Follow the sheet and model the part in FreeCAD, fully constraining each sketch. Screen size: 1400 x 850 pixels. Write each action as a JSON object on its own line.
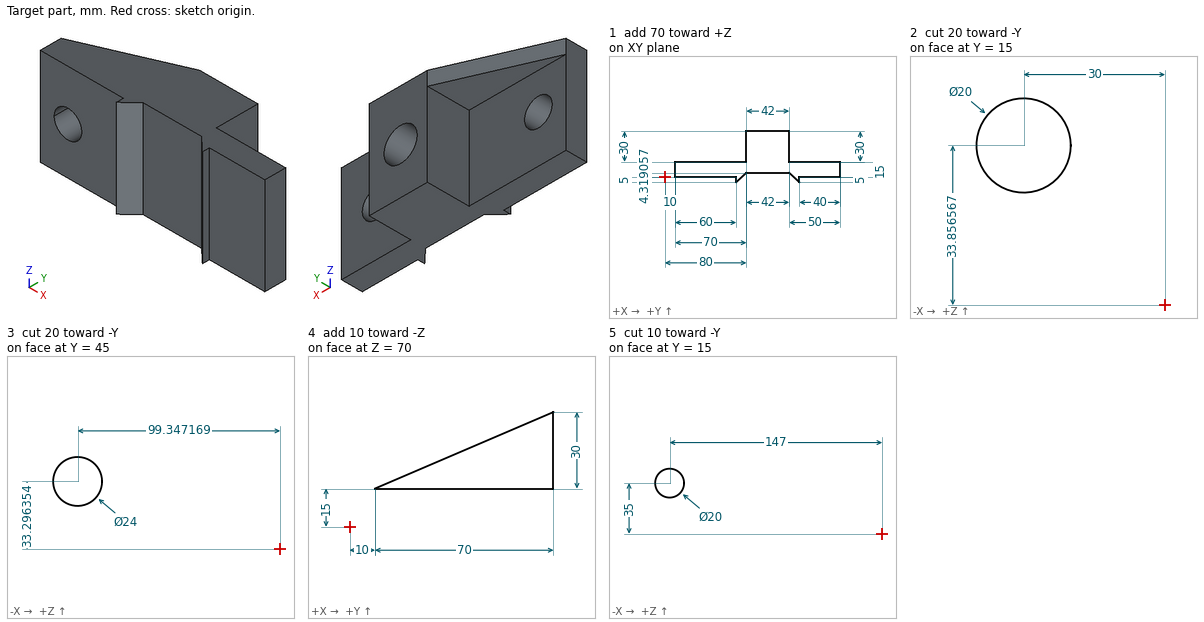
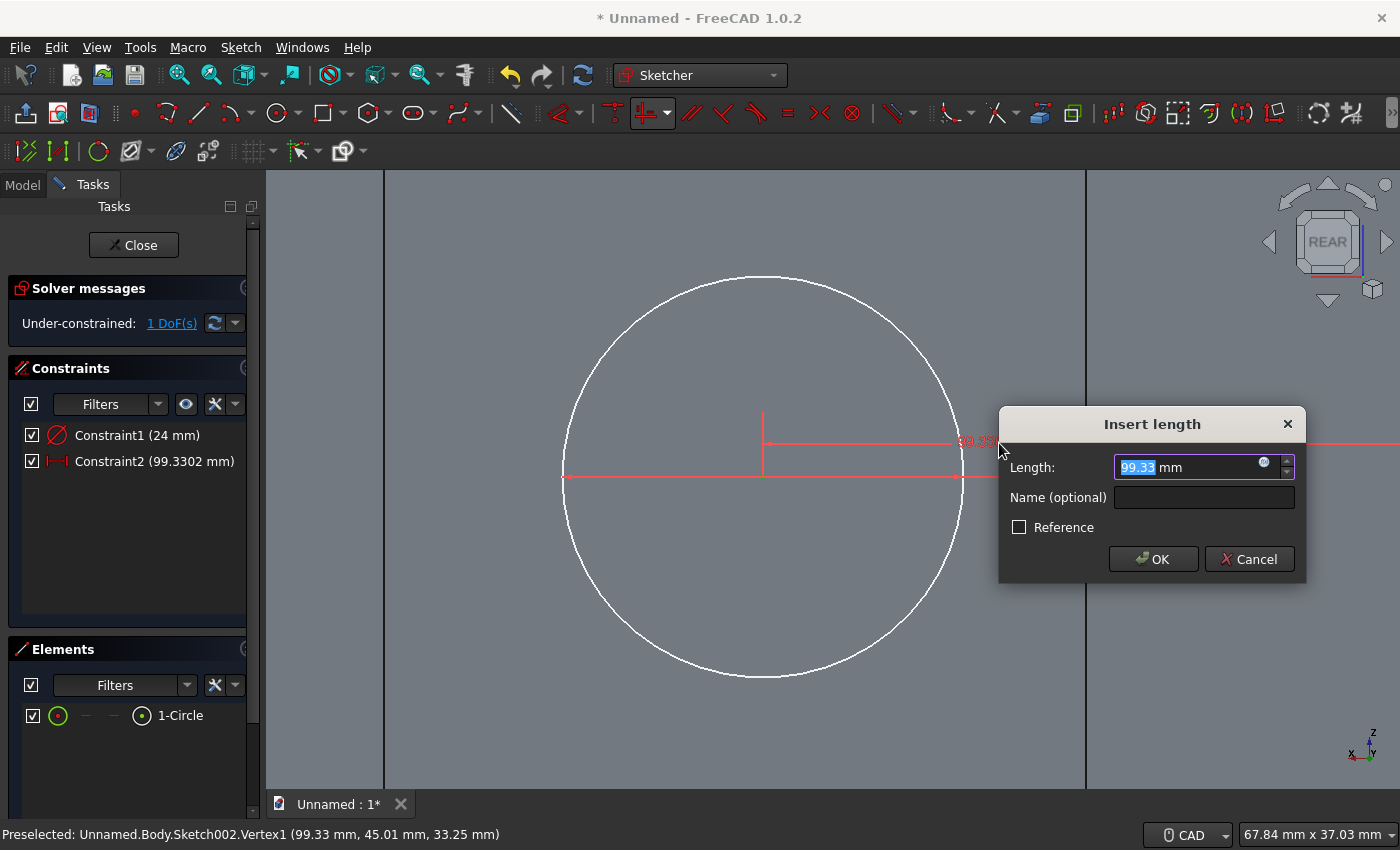
{"action": "type", "text": "99.347169"}
{"action": "key", "text": "Return"}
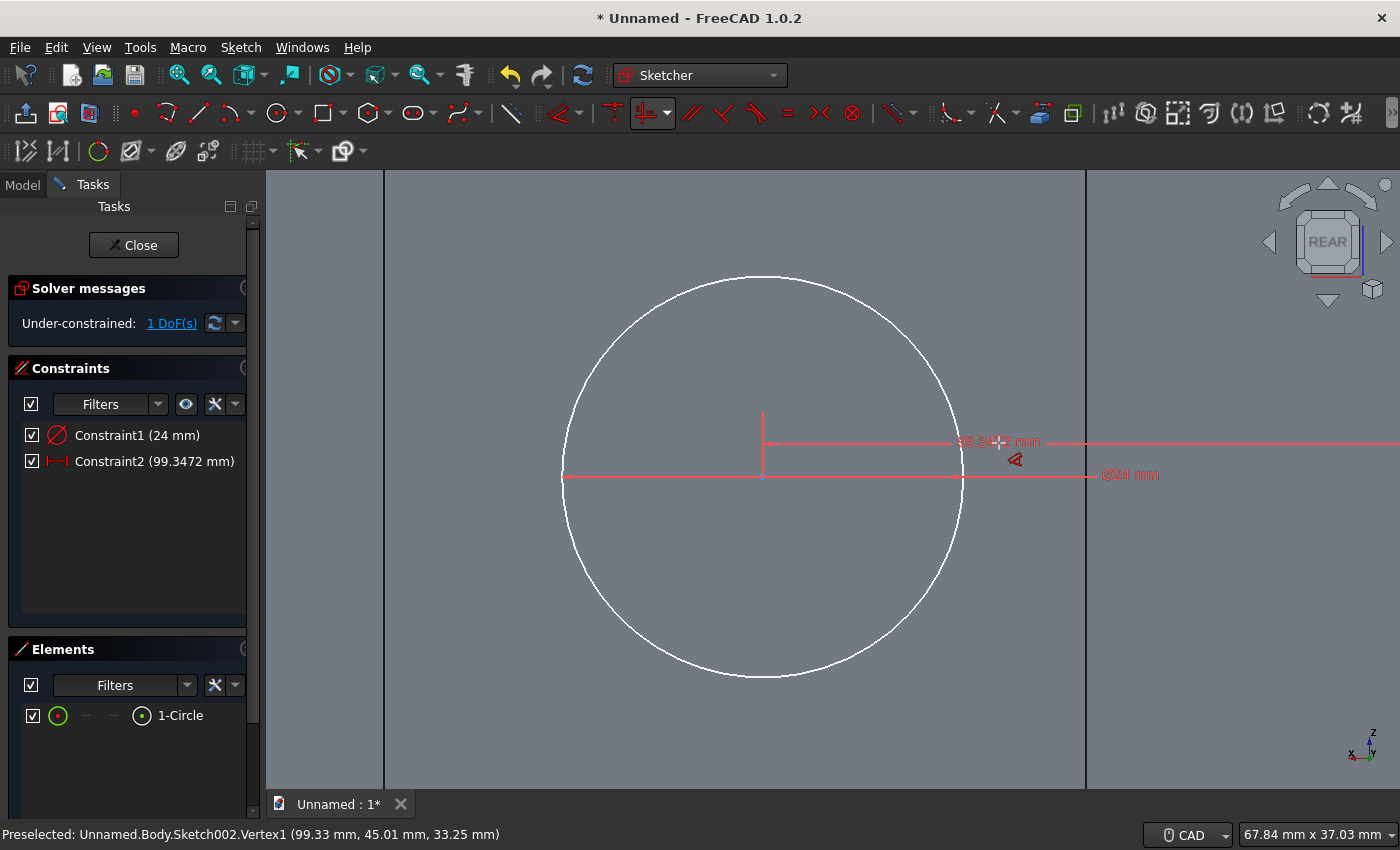
{"action": "left_click", "coordinate": [763, 477]}
{"action": "left_click", "coordinate": [729, 619]}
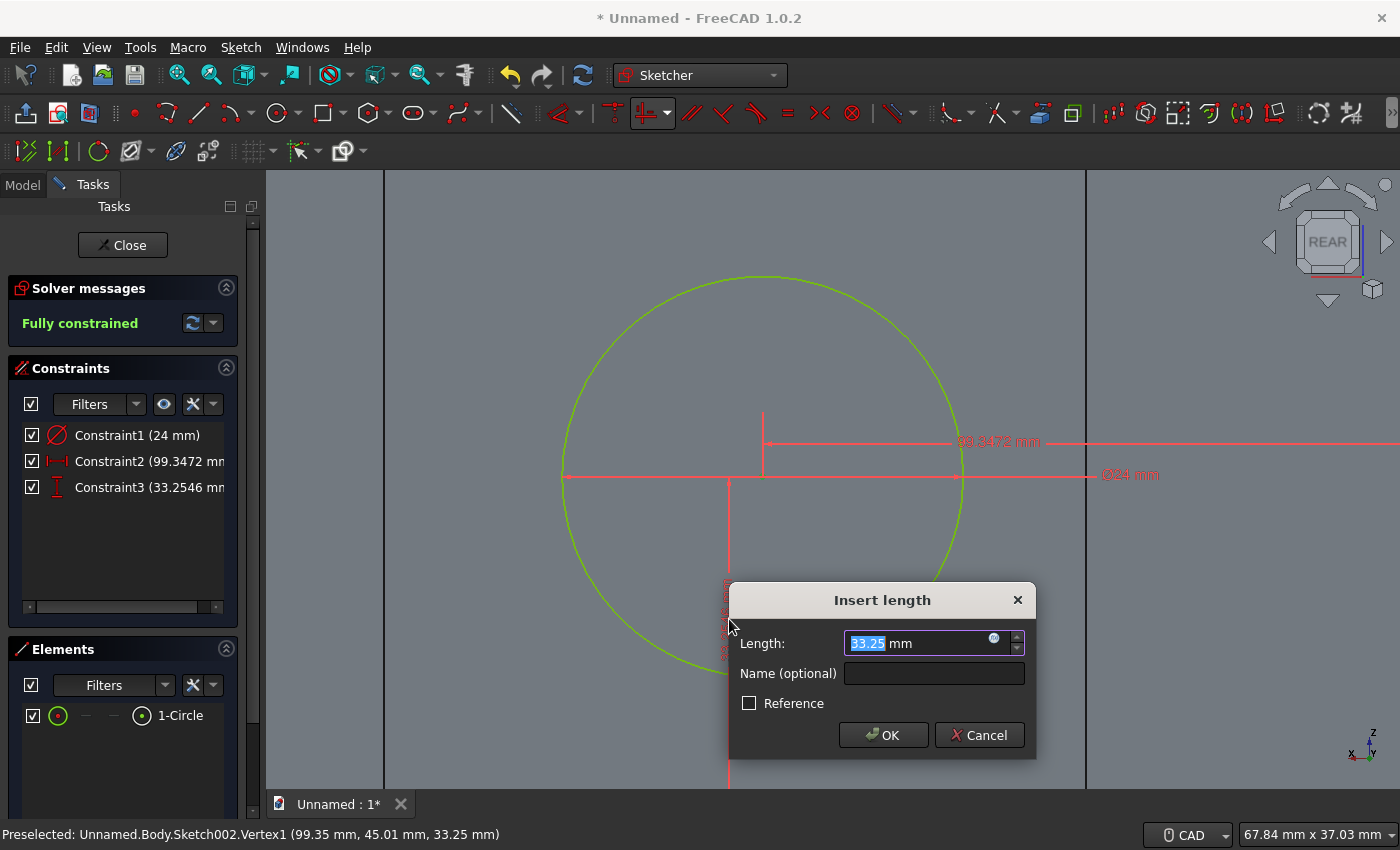
{"action": "type", "text": "33.296354"}
{"action": "key", "text": "Return"}
{"action": "key", "text": "Escape"}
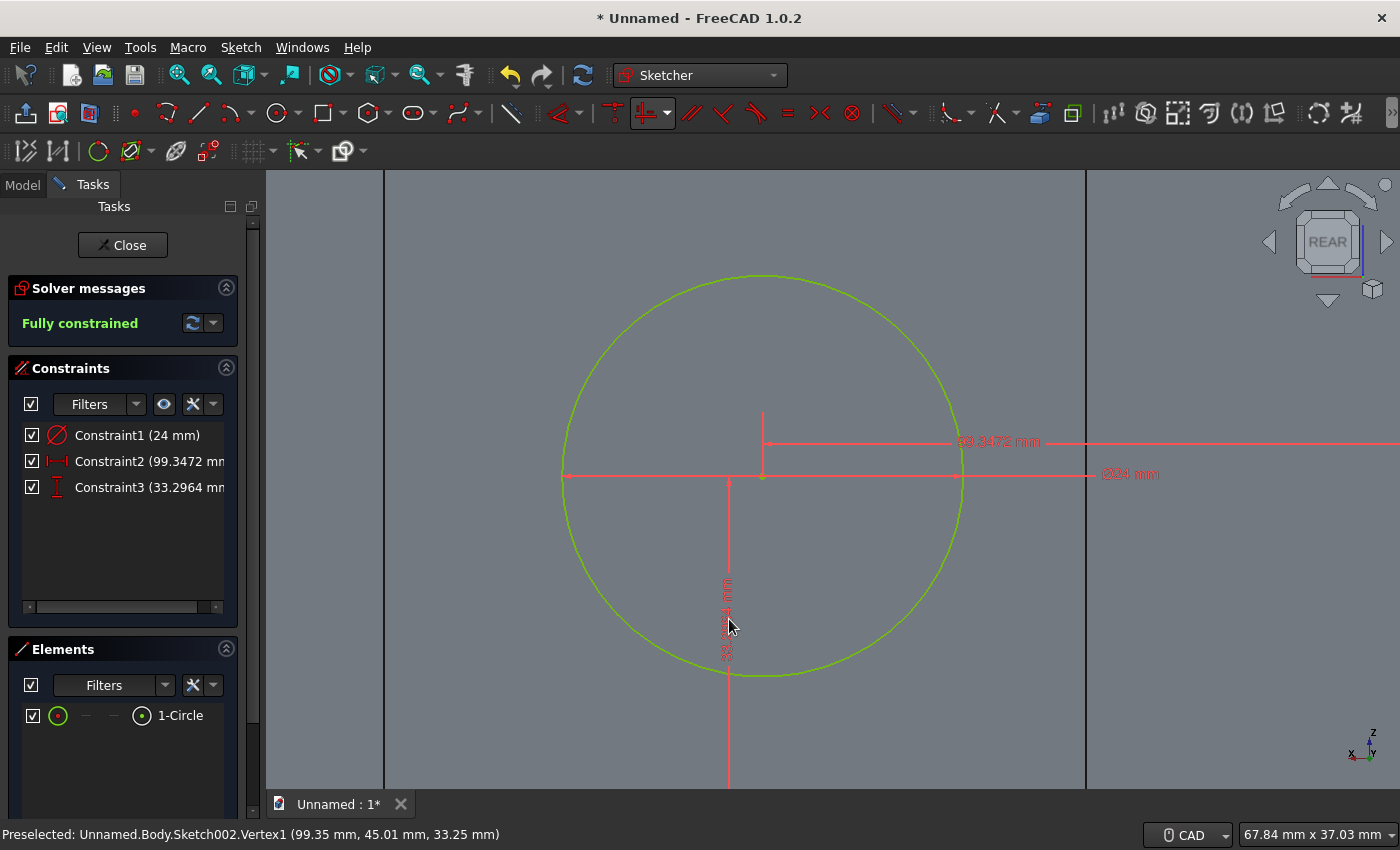
{"action": "left_click", "coordinate": [123, 245]}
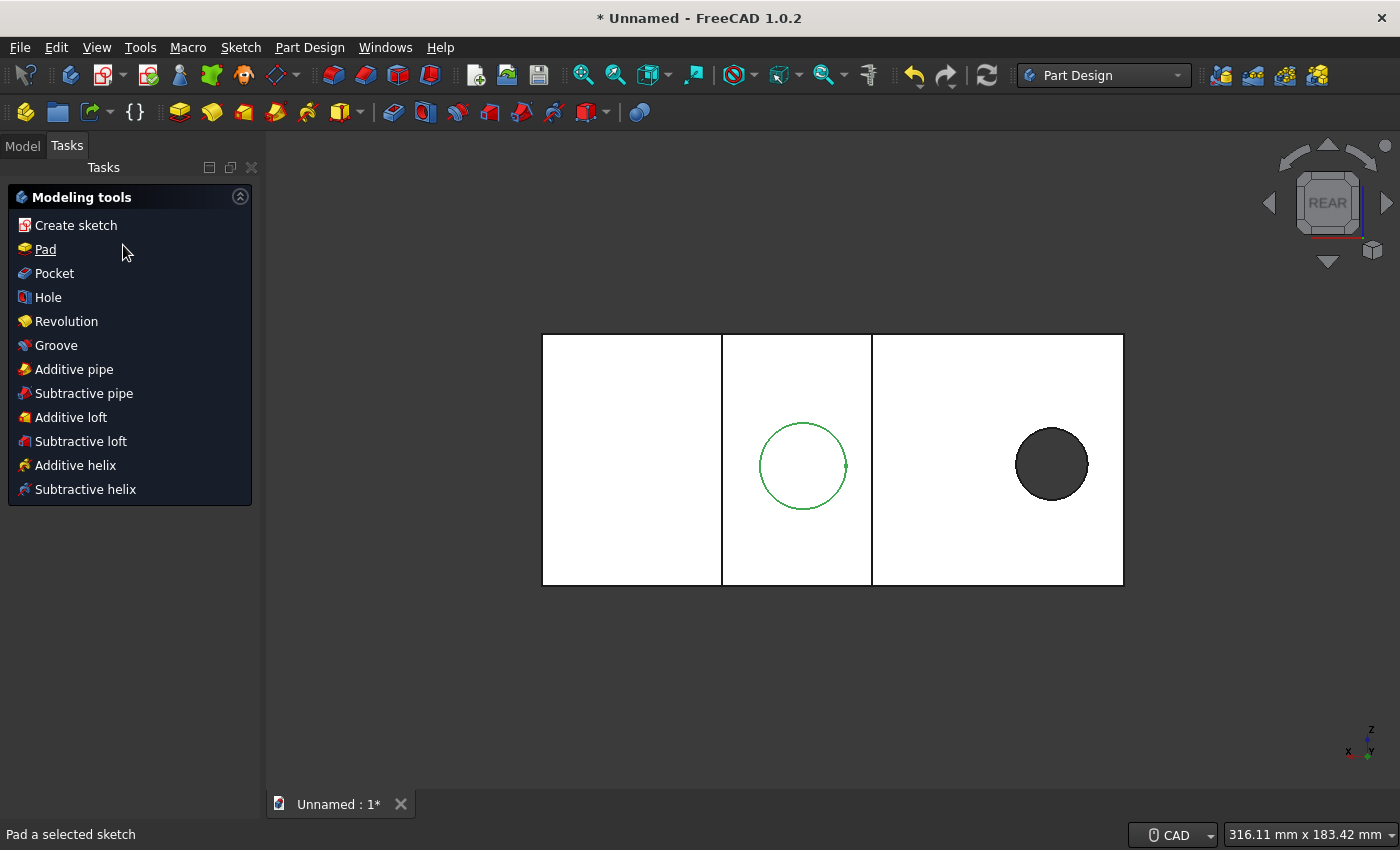
{"action": "left_click", "coordinate": [394, 112]}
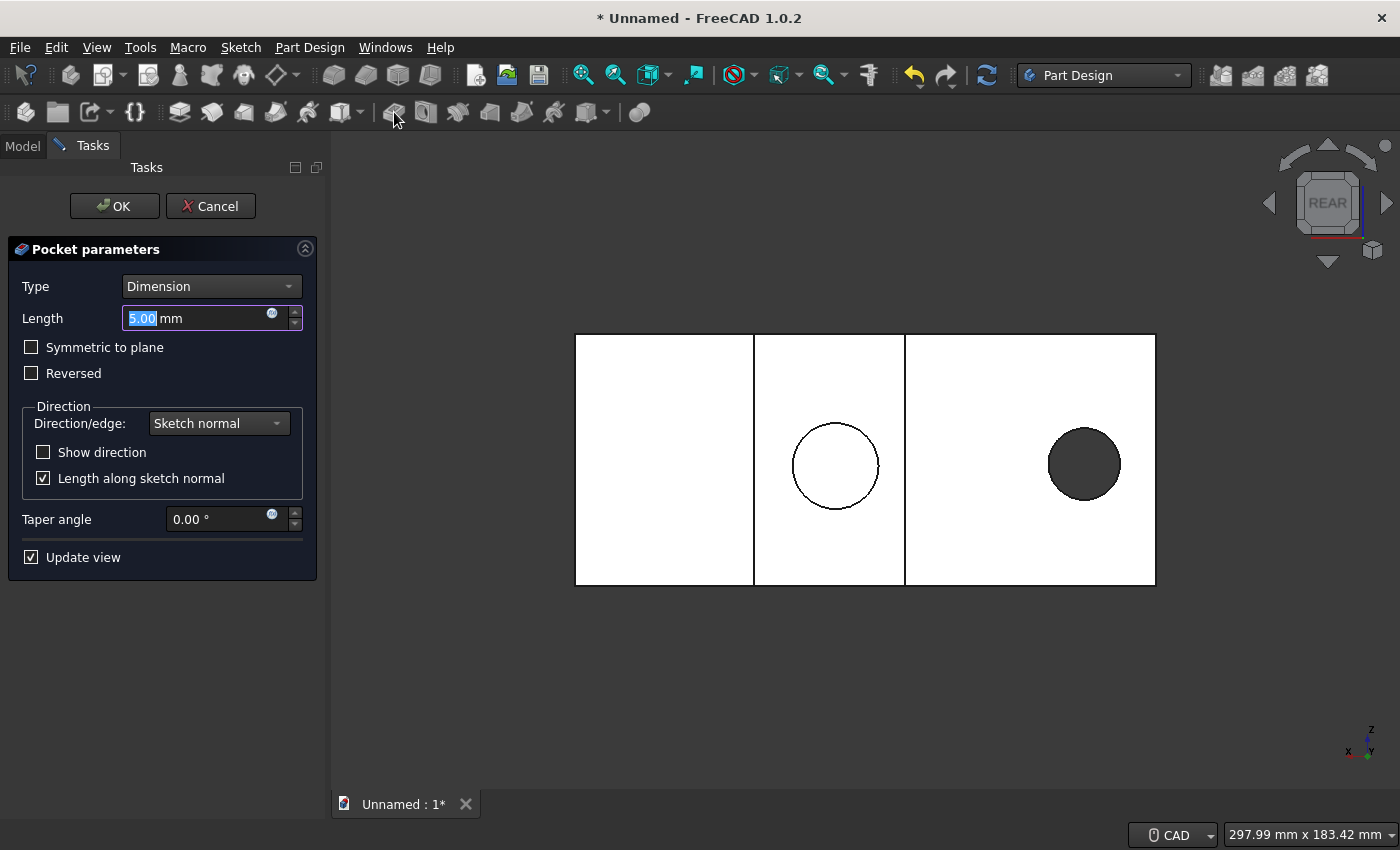
{"action": "type", "text": "20"}
{"action": "key", "text": "Tab"}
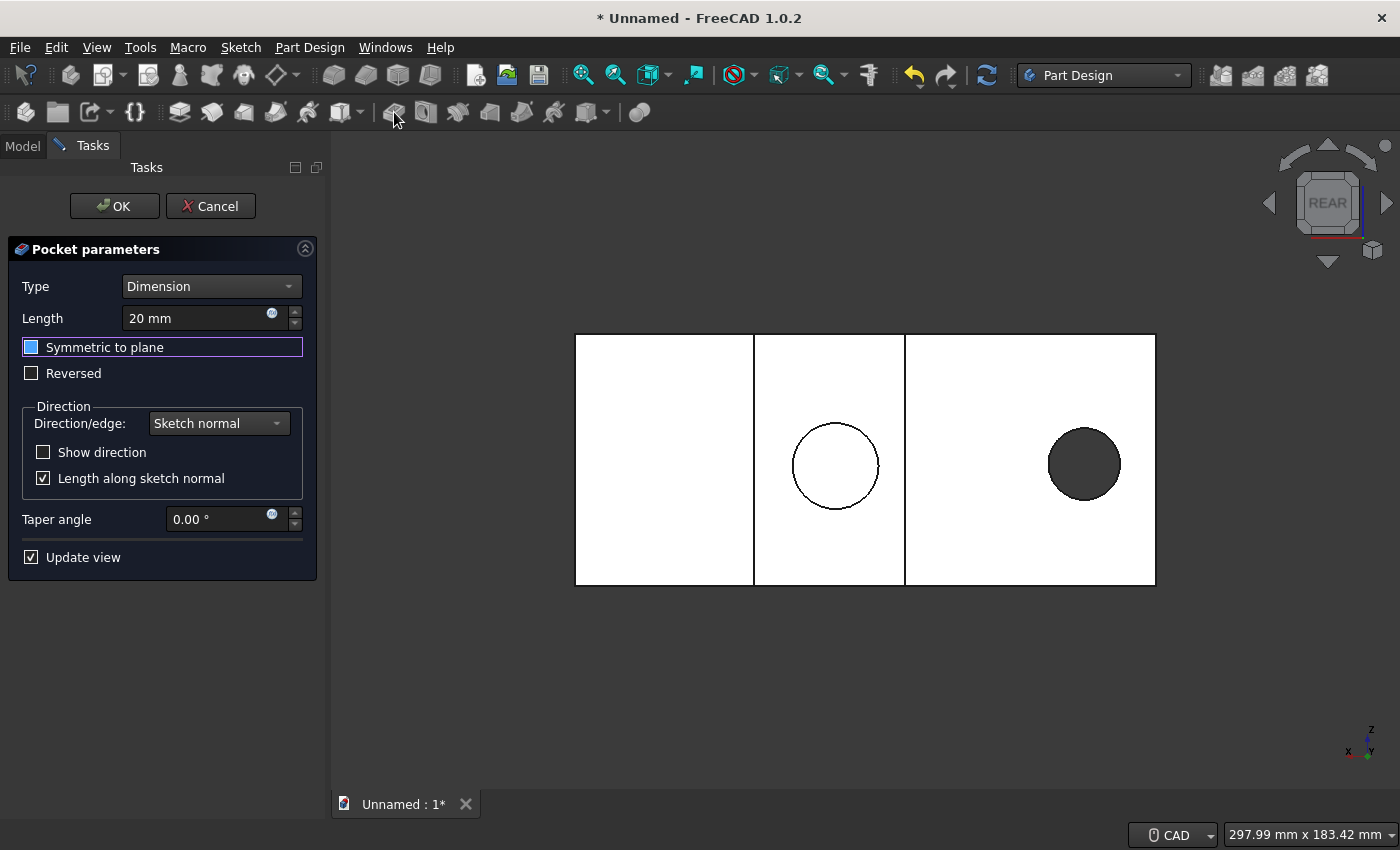
{"action": "left_click", "coordinate": [115, 206]}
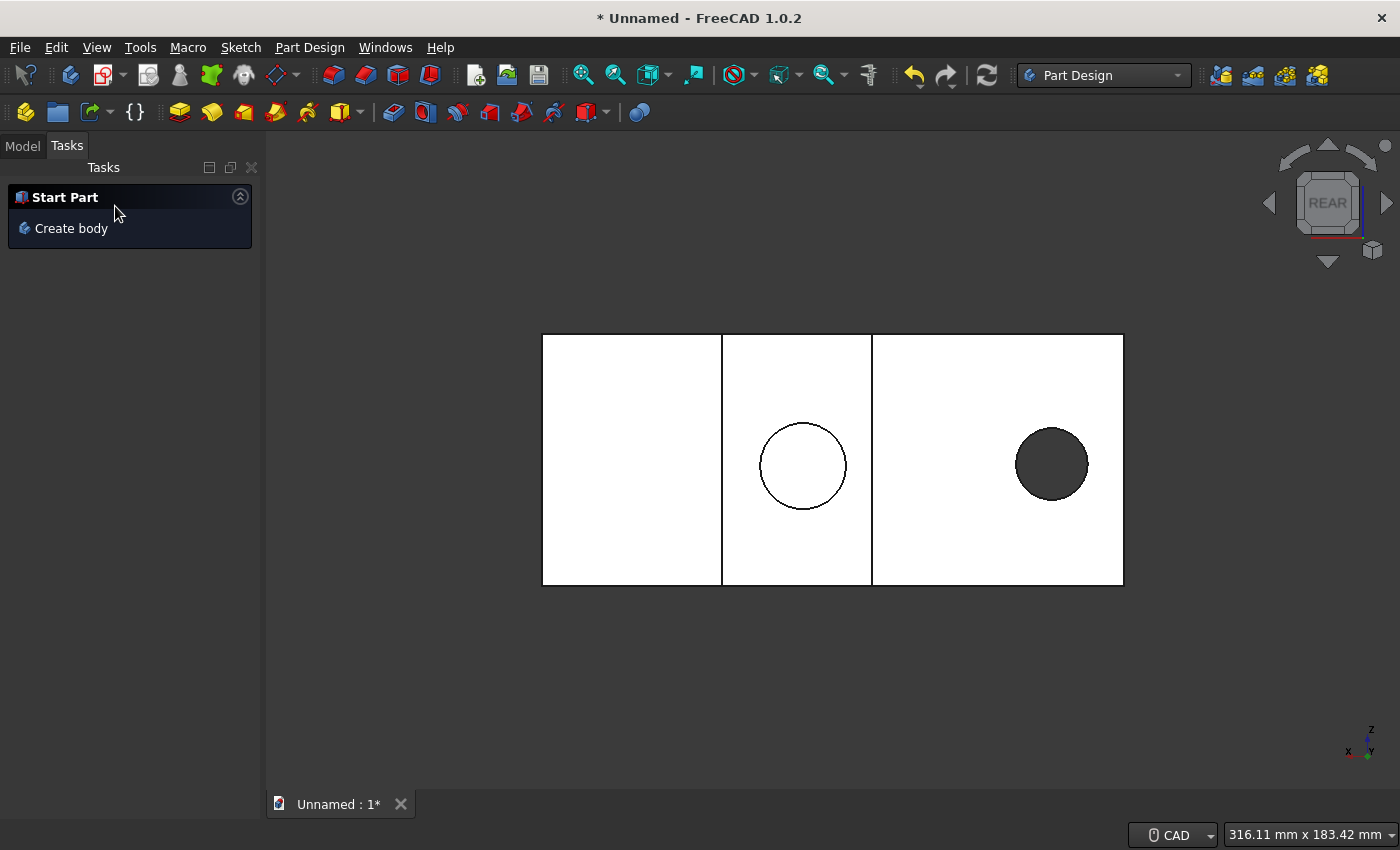
{"action": "key", "text": "0"}